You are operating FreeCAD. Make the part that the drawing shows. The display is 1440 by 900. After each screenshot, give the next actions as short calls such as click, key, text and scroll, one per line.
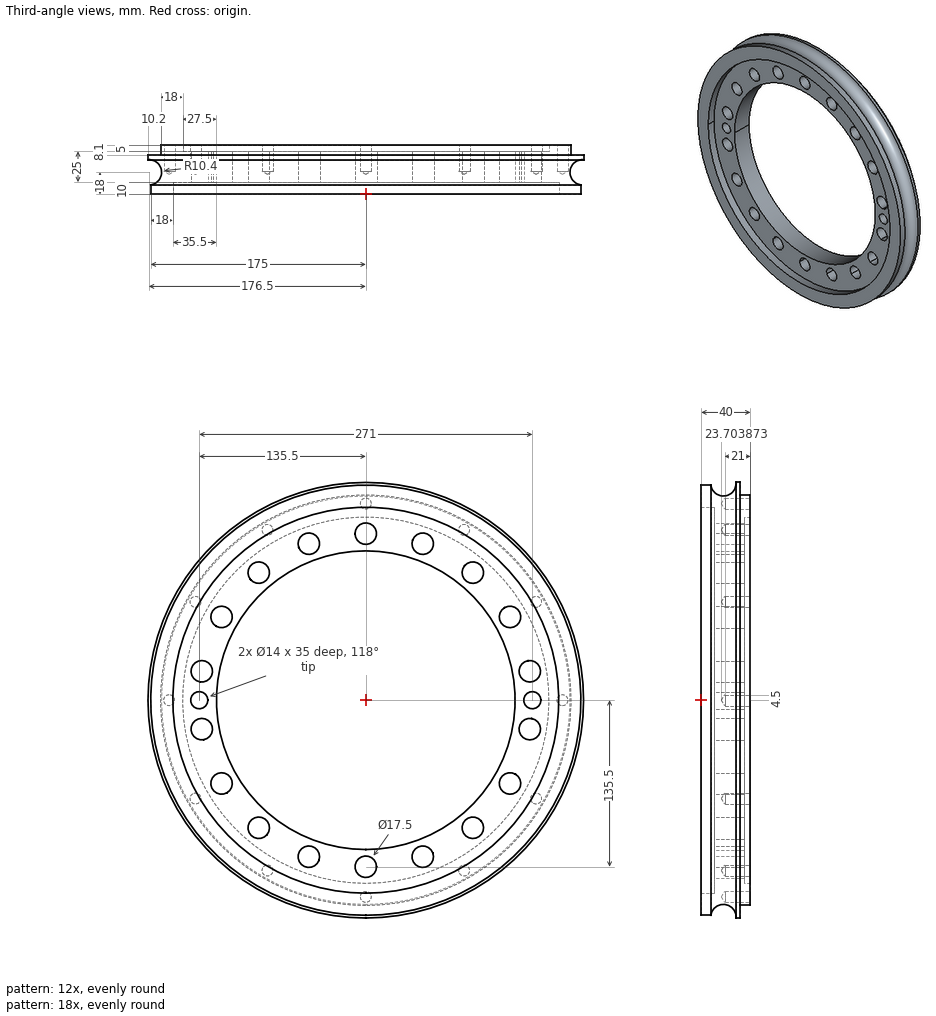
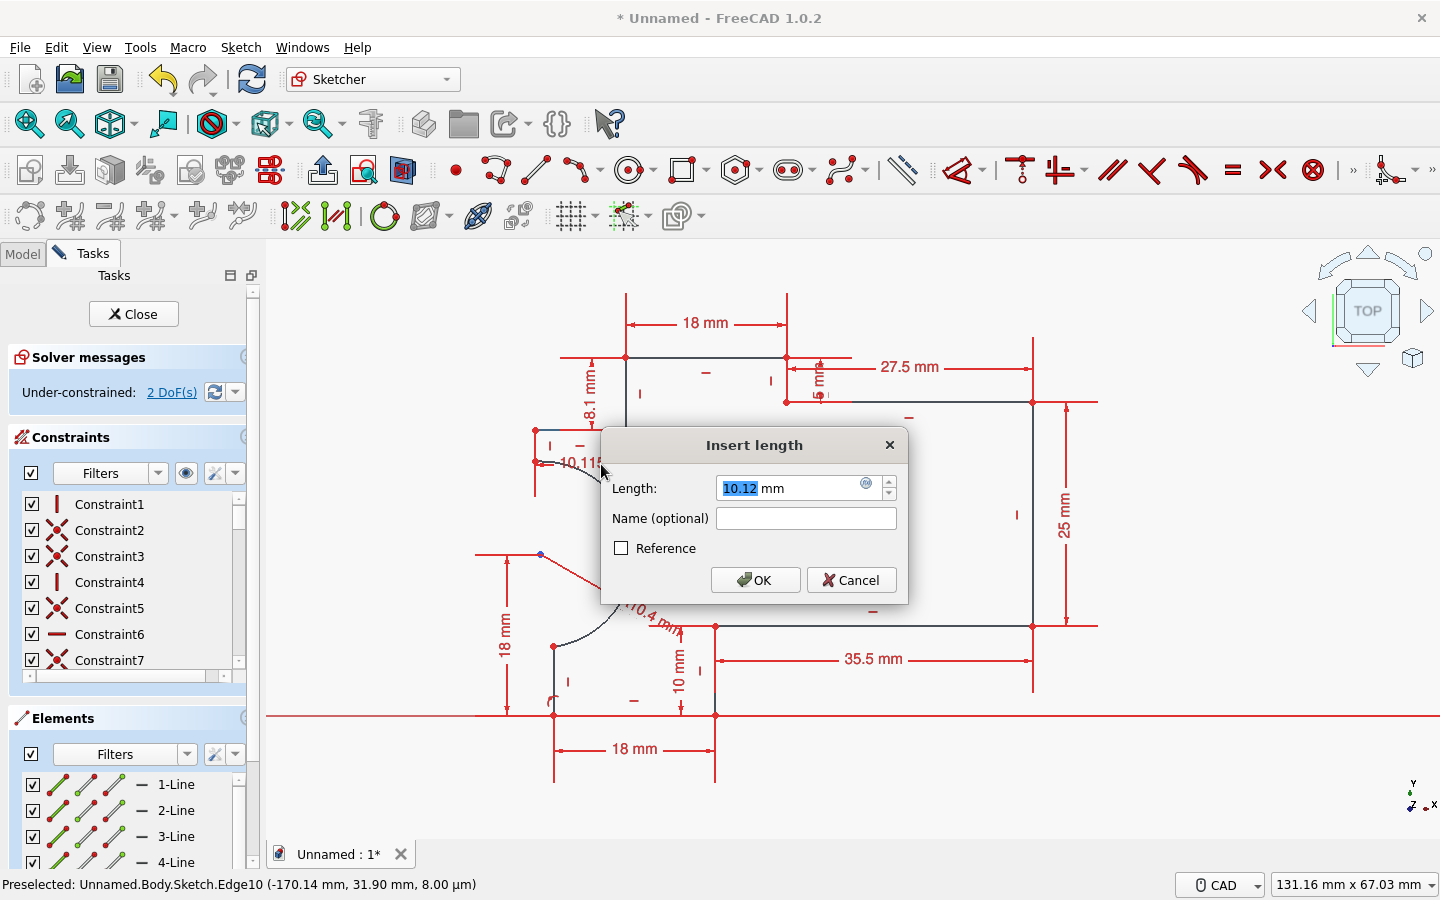
text(10.2)
key(Return)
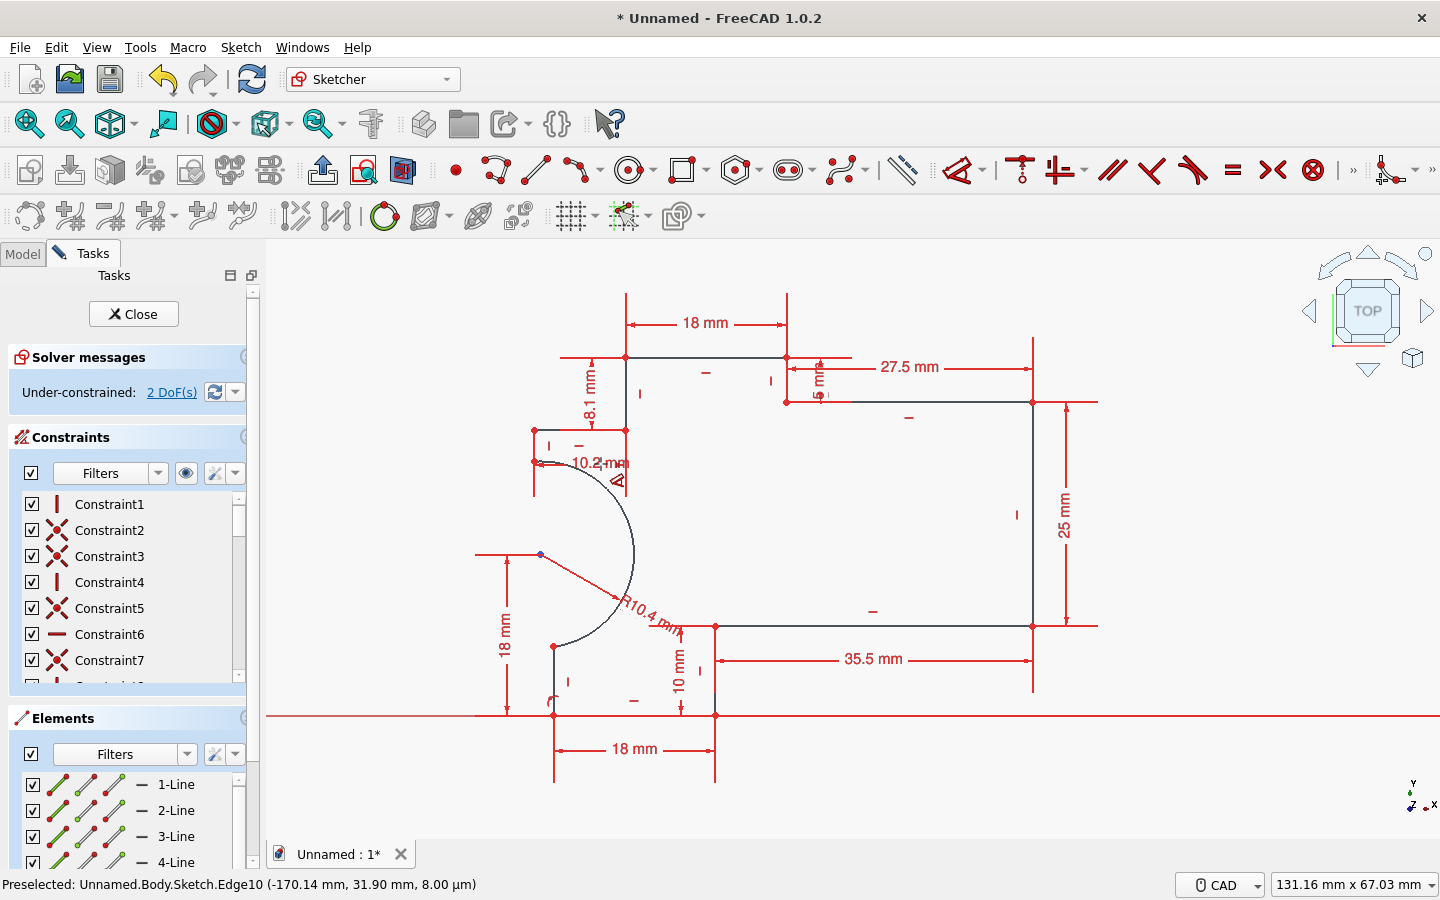
click(554, 647)
click(914, 750)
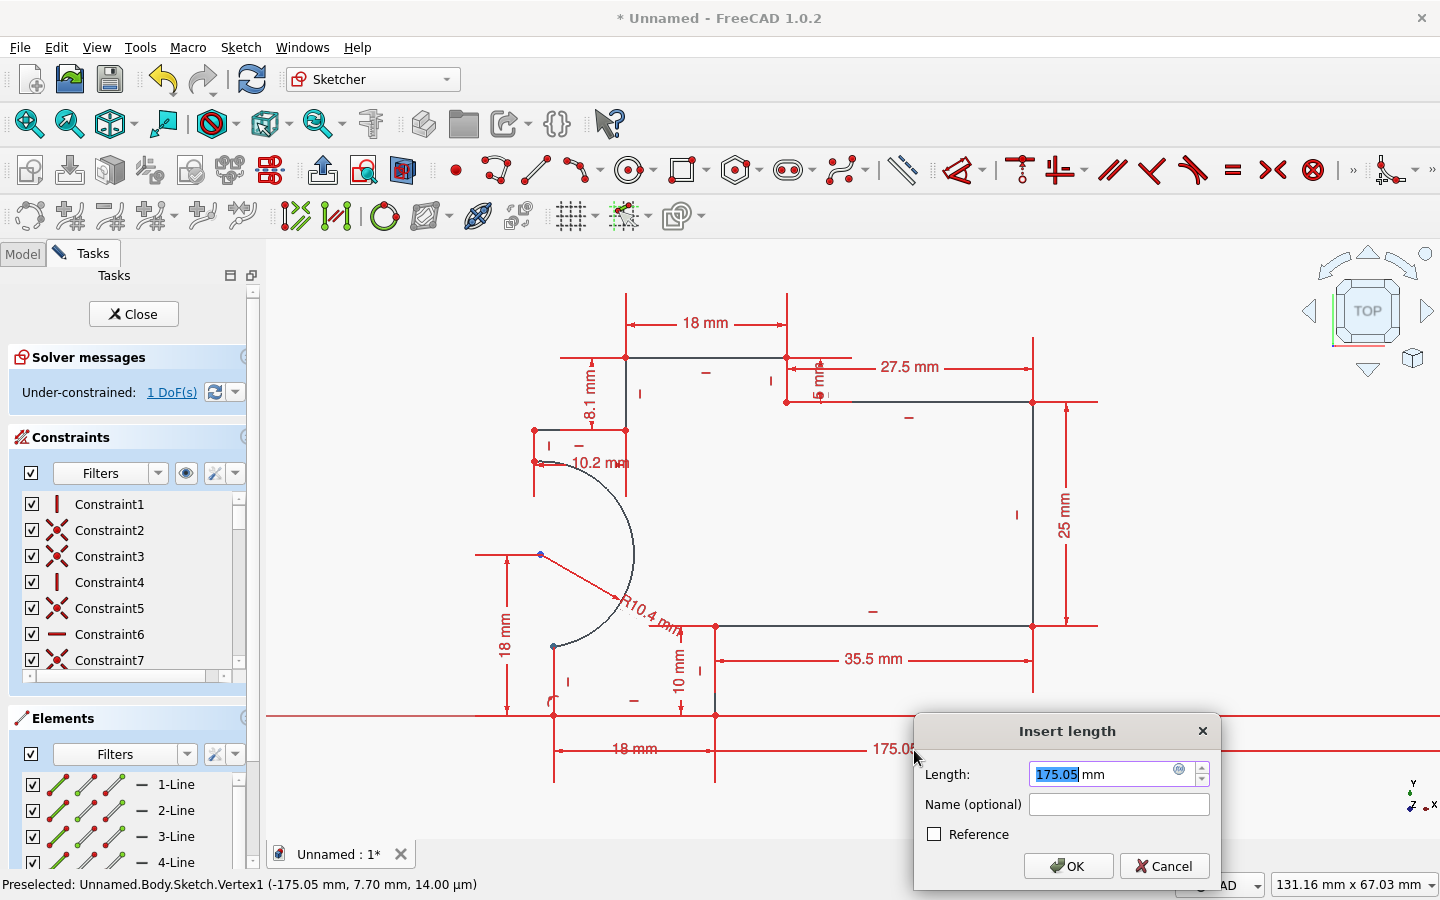
text(175)
key(Return)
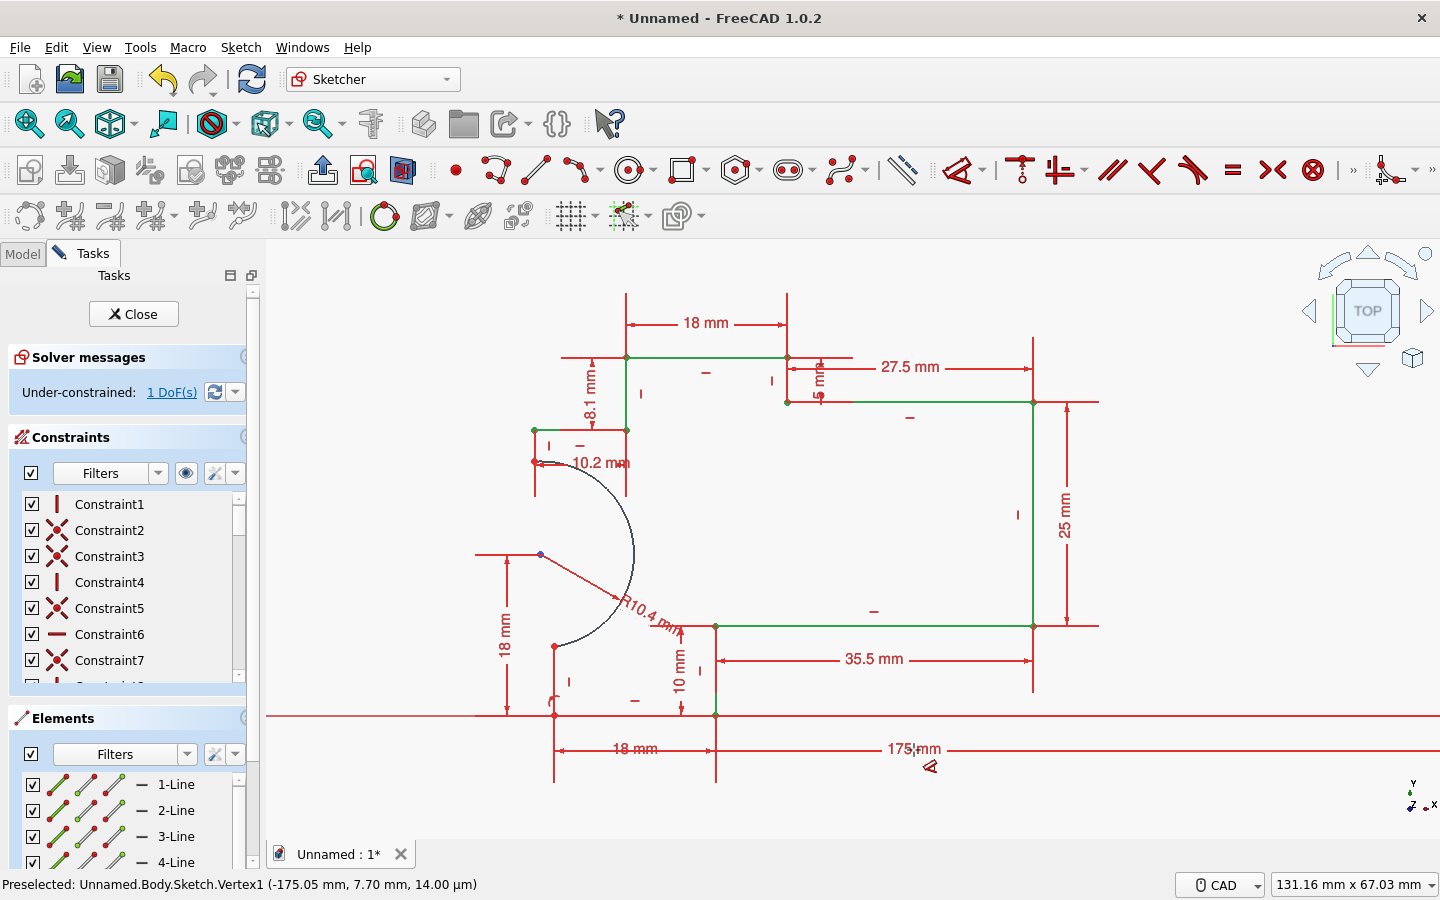
click(541, 555)
click(739, 750)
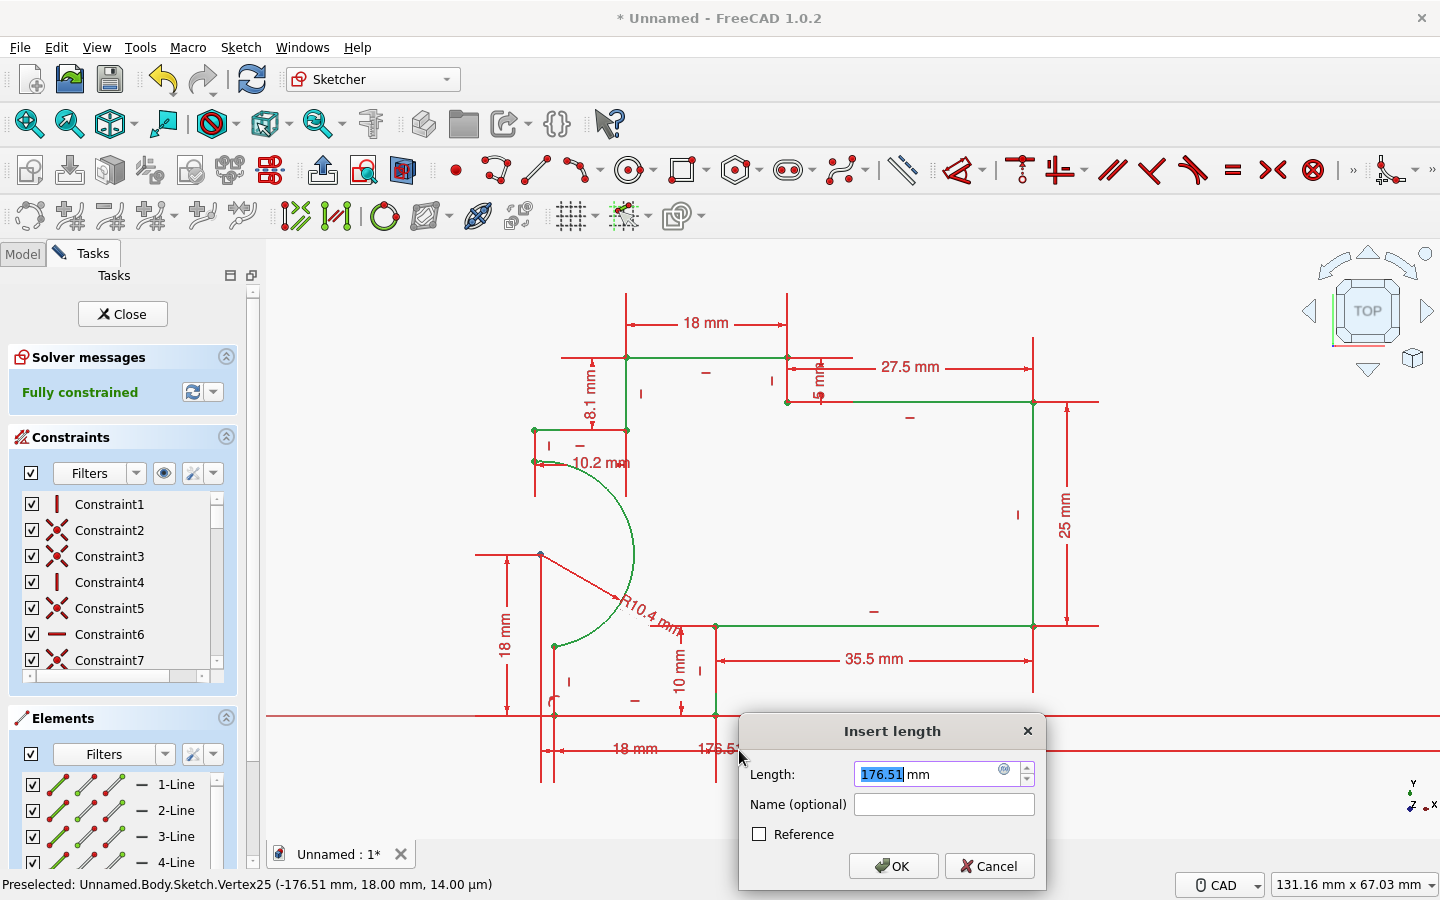
text(176.5)
key(Return)
key(Escape)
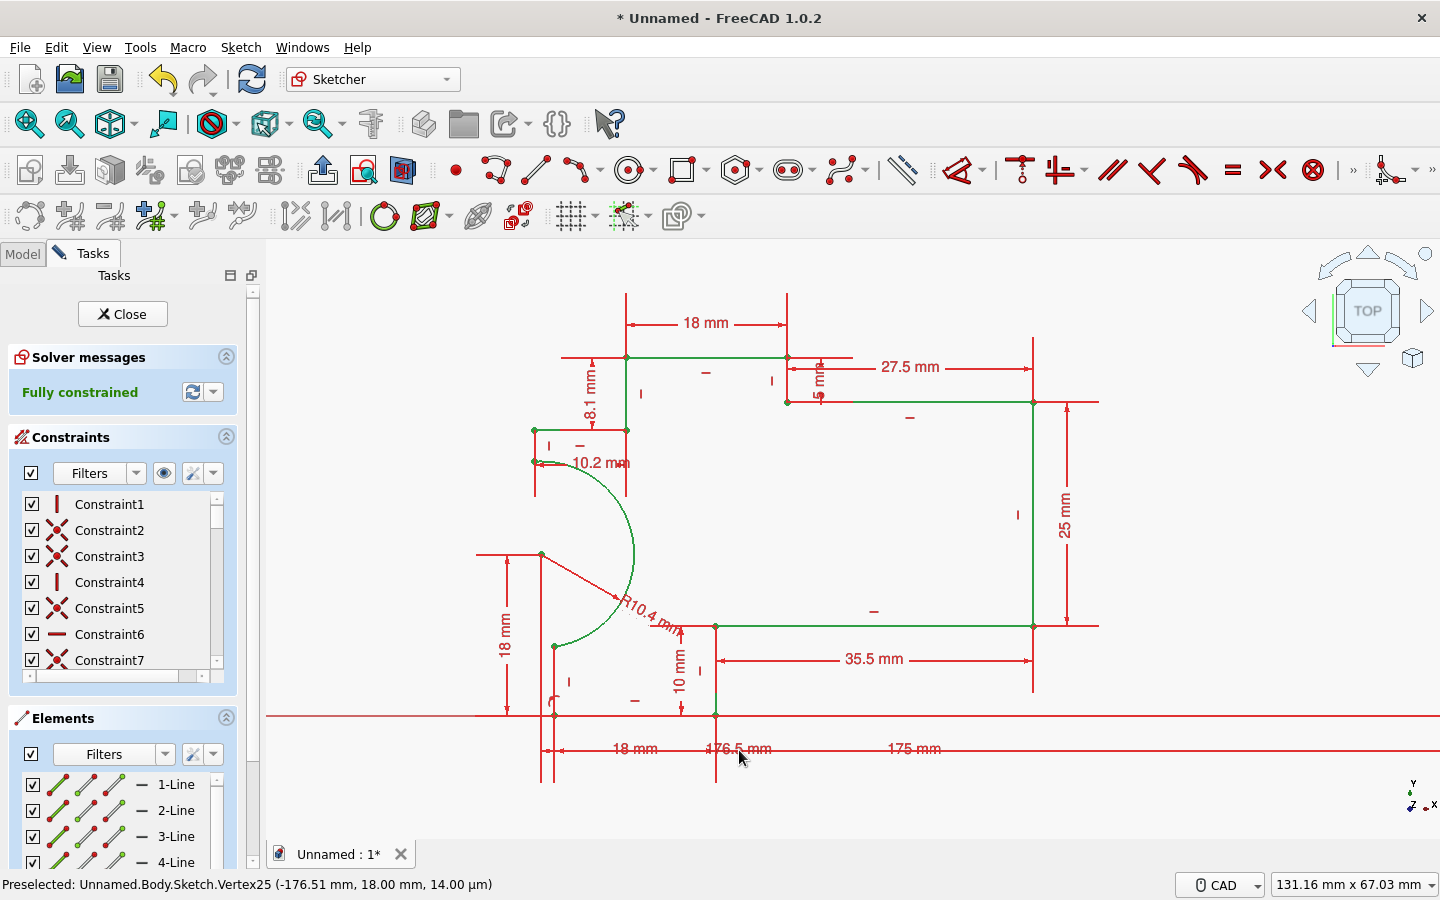
click(123, 314)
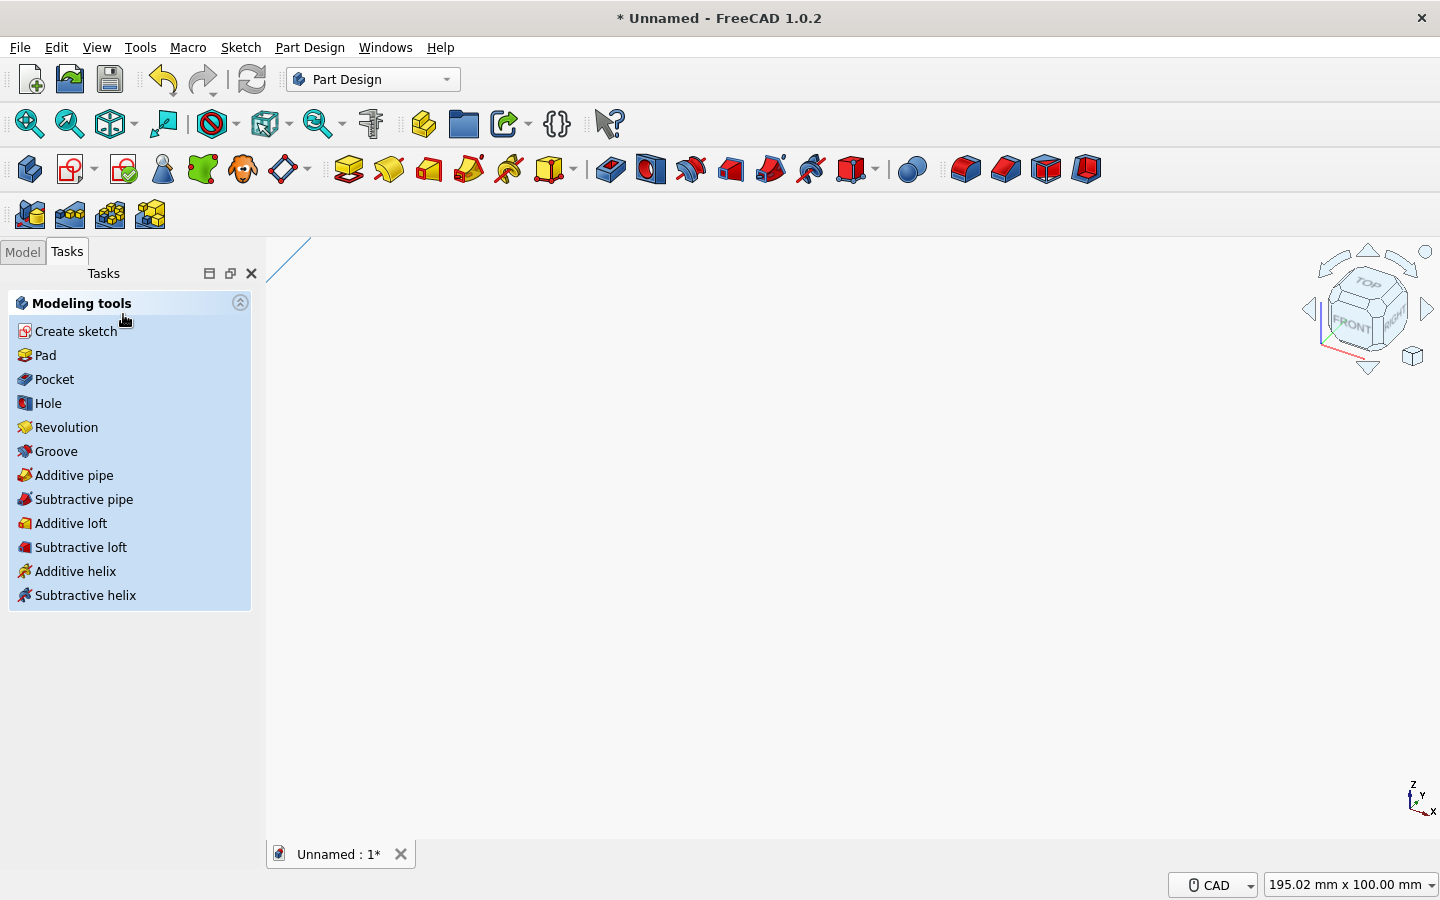
click(390, 170)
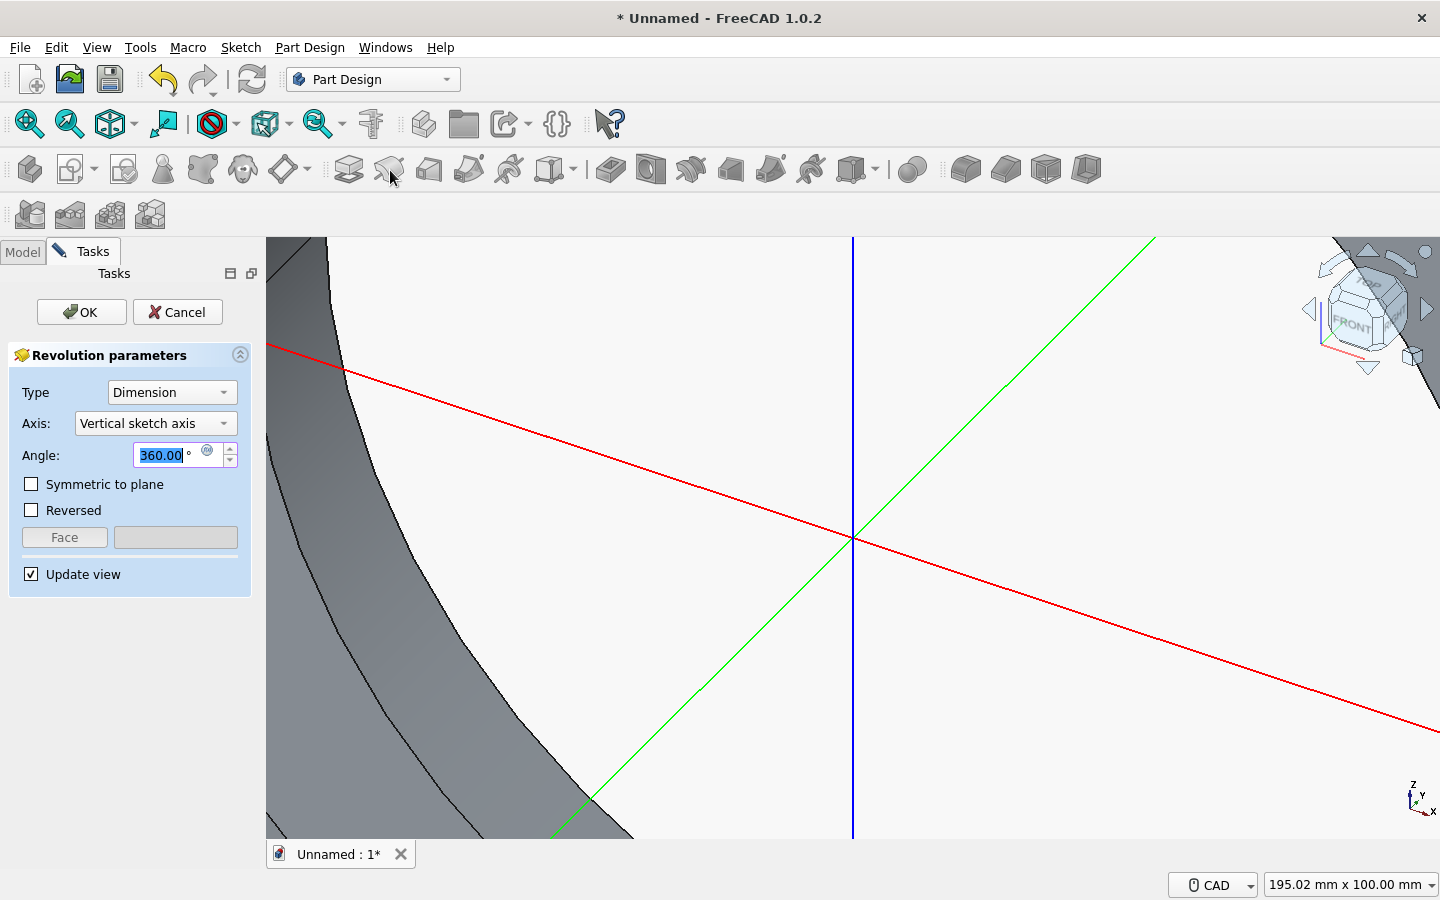
click(82, 312)